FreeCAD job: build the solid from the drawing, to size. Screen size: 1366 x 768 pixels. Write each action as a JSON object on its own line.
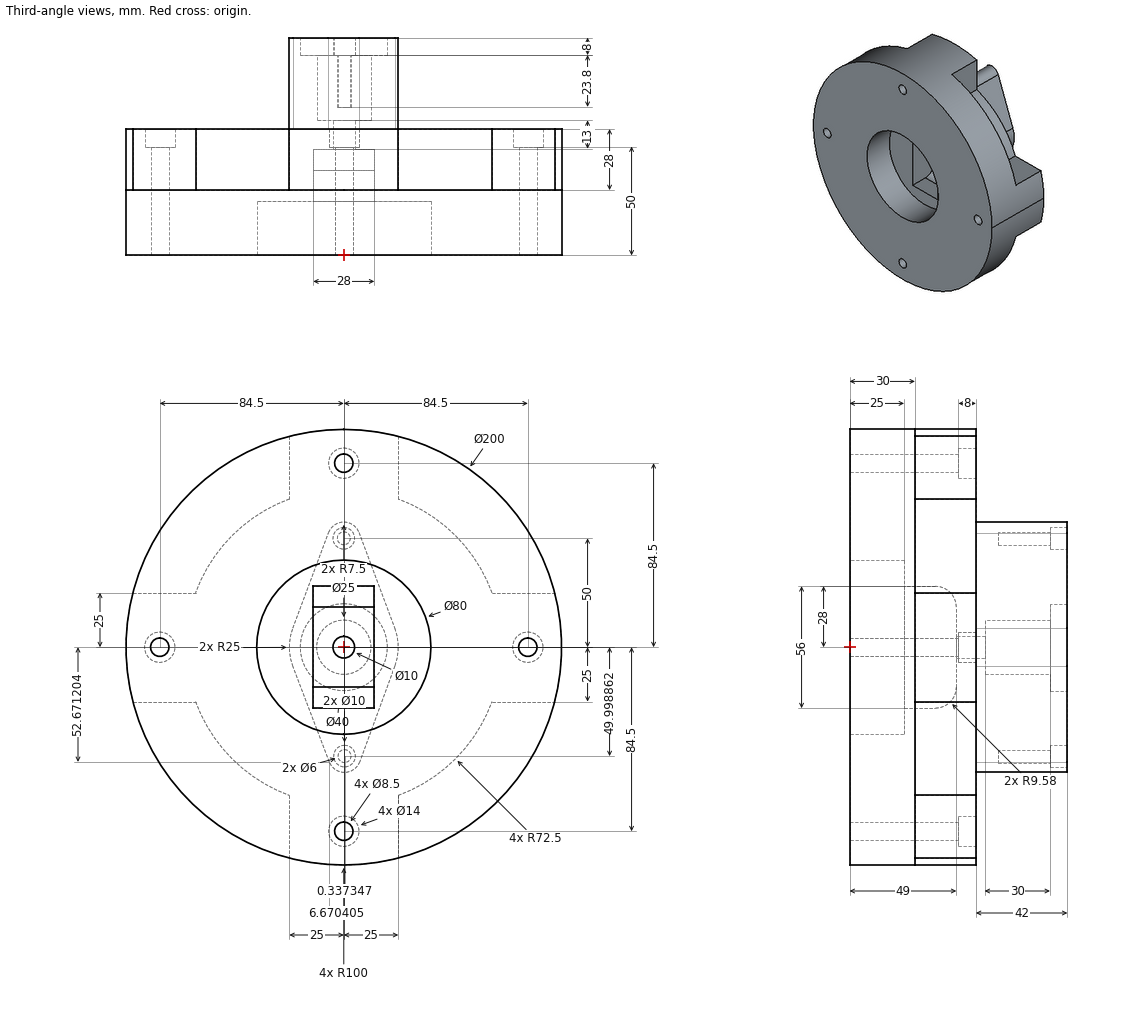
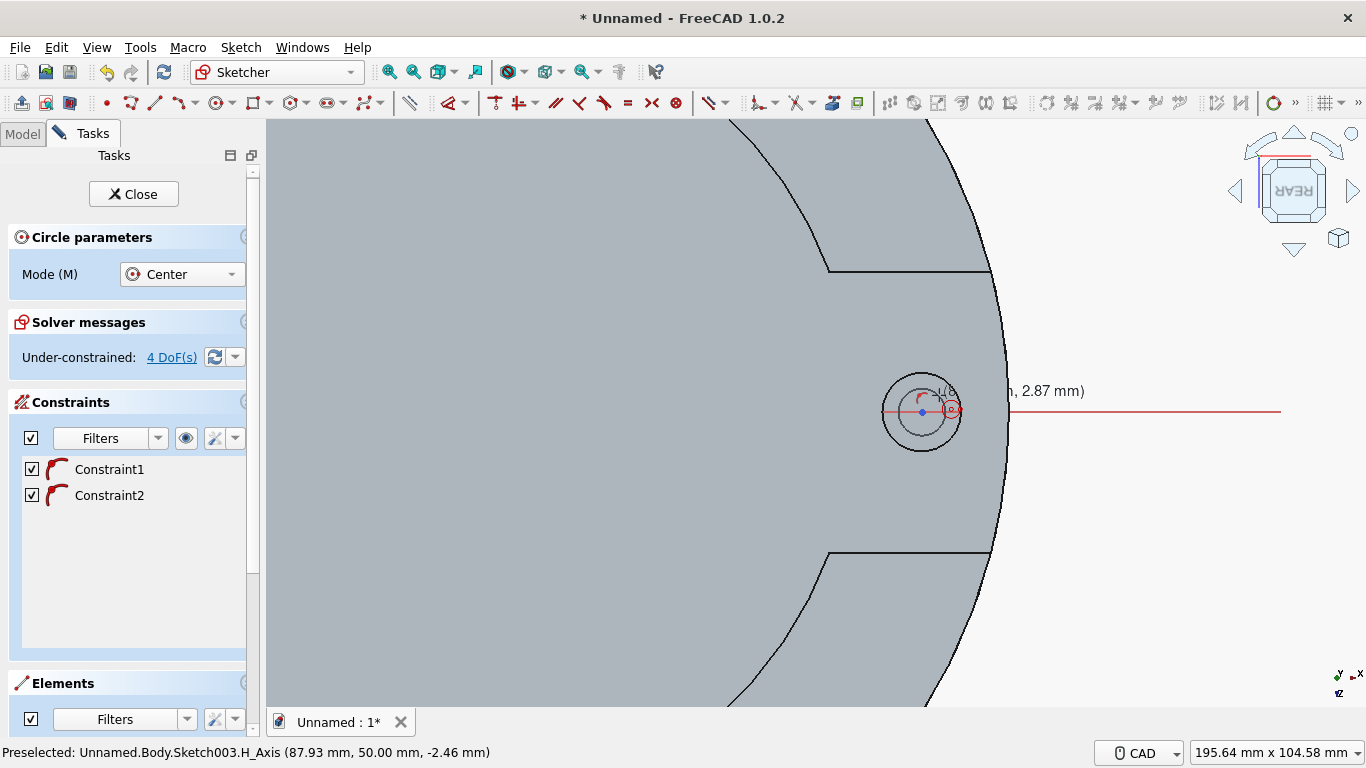
{"action": "scroll", "coordinate": [923, 414], "scroll_direction": "down", "scroll_amount": 5}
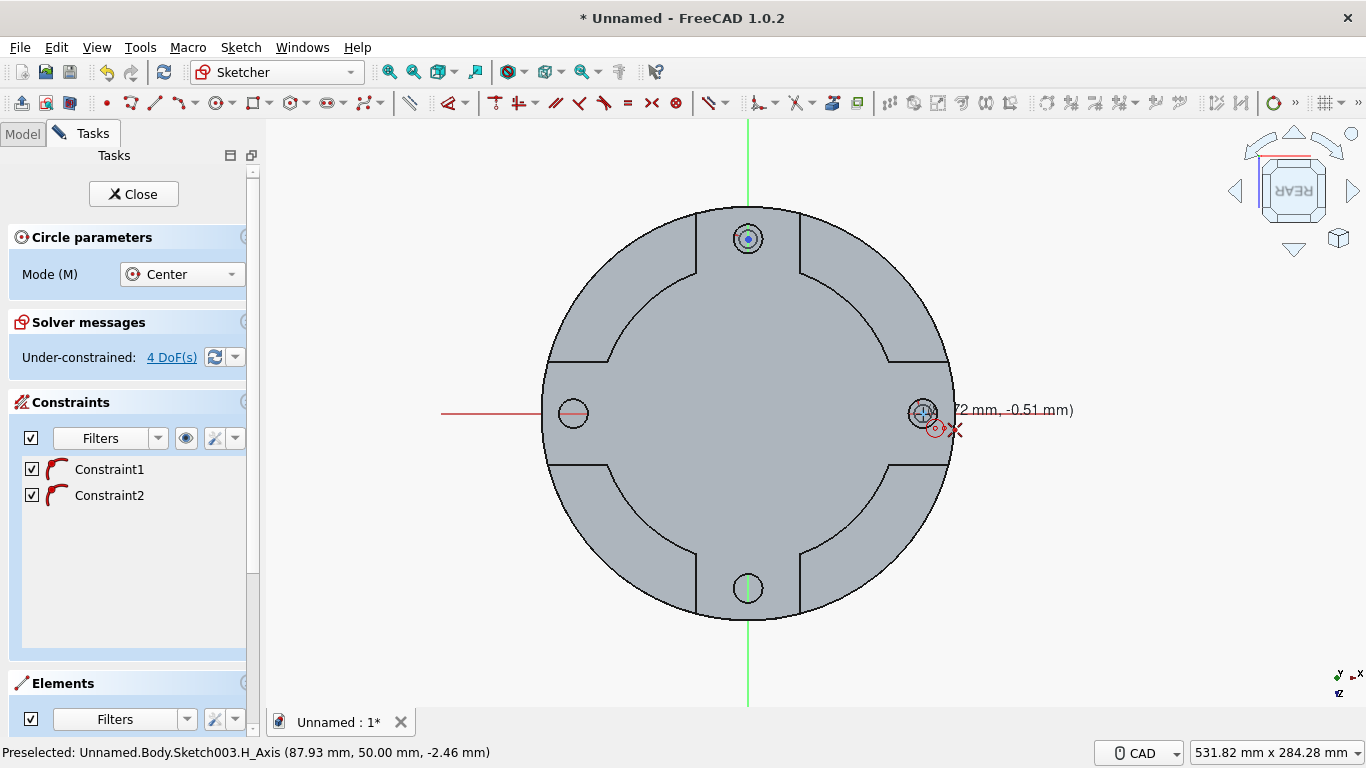
{"action": "scroll", "coordinate": [748, 588], "scroll_direction": "up", "scroll_amount": 5}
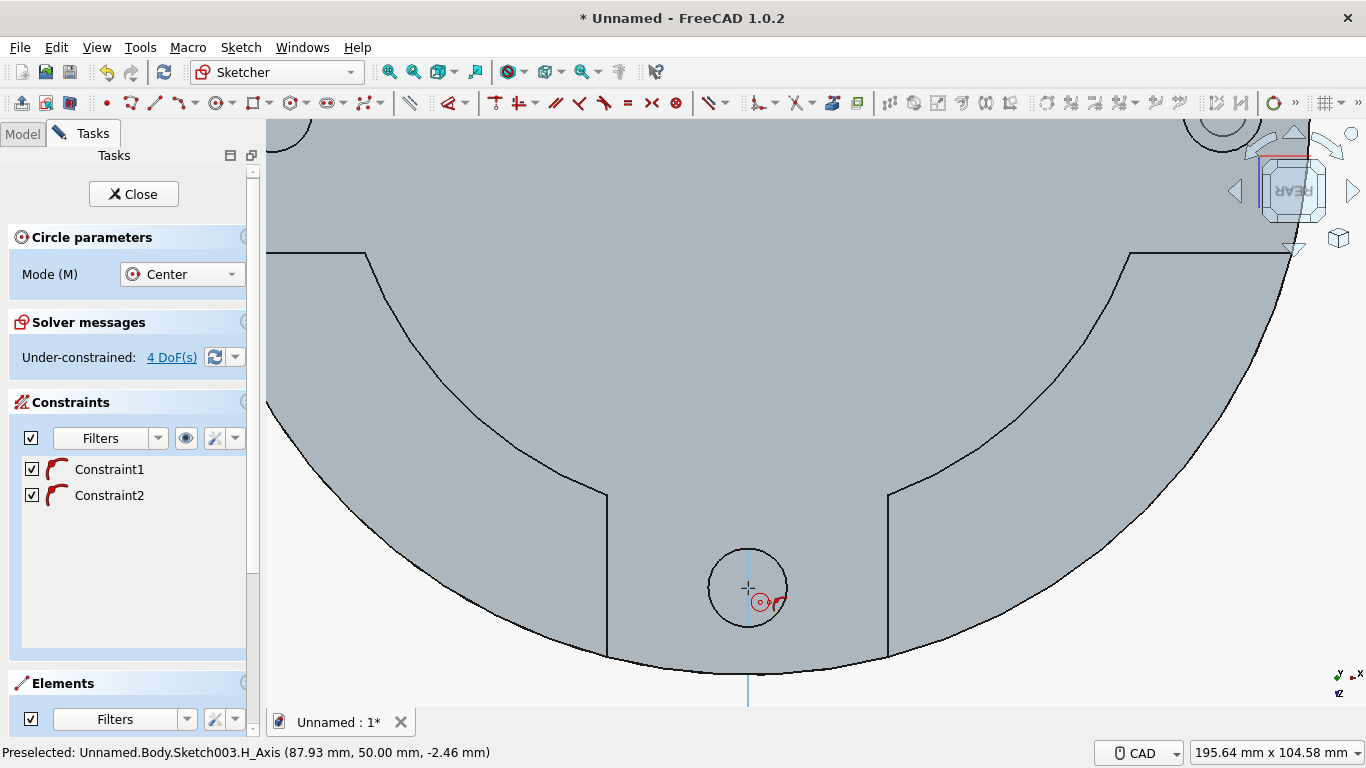
{"action": "left_click", "coordinate": [748, 588]}
{"action": "left_click", "coordinate": [765, 571]}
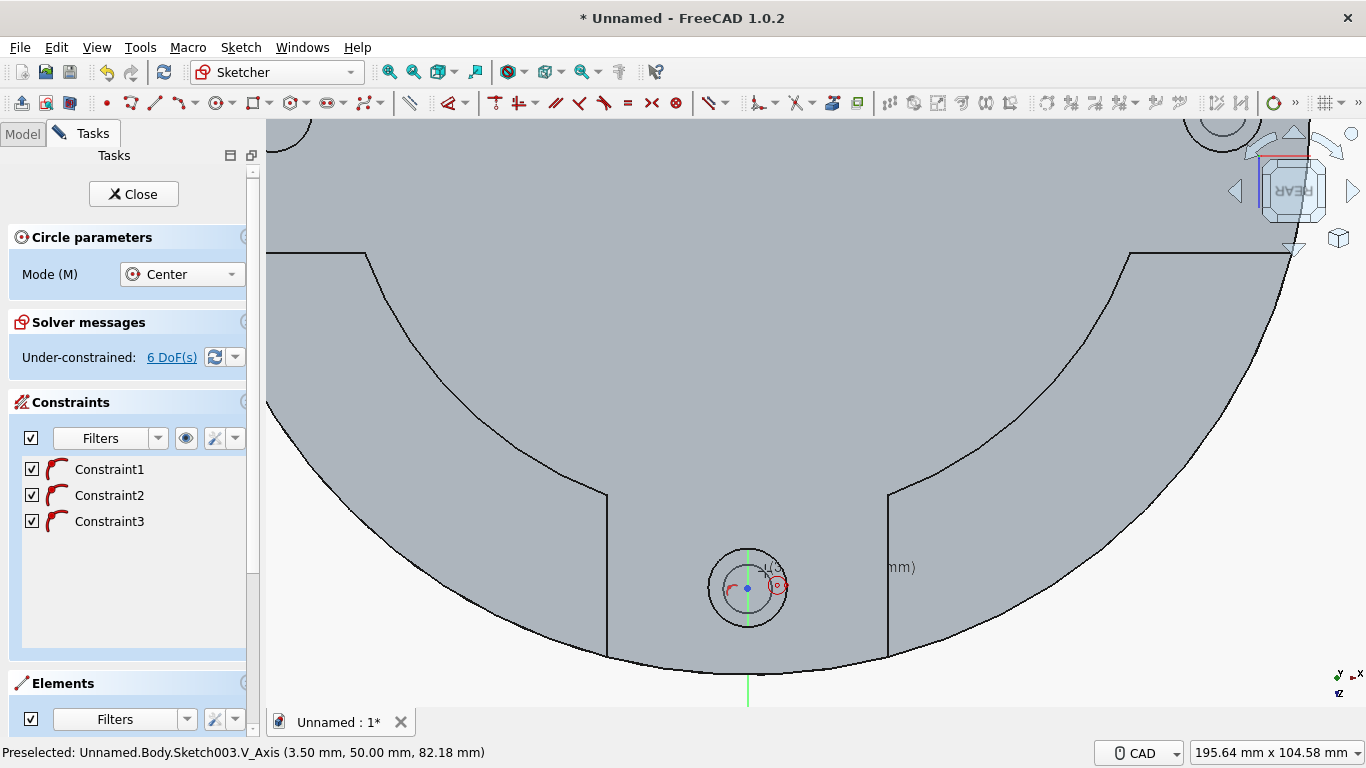
{"action": "scroll", "coordinate": [747, 588], "scroll_direction": "down", "scroll_amount": 5}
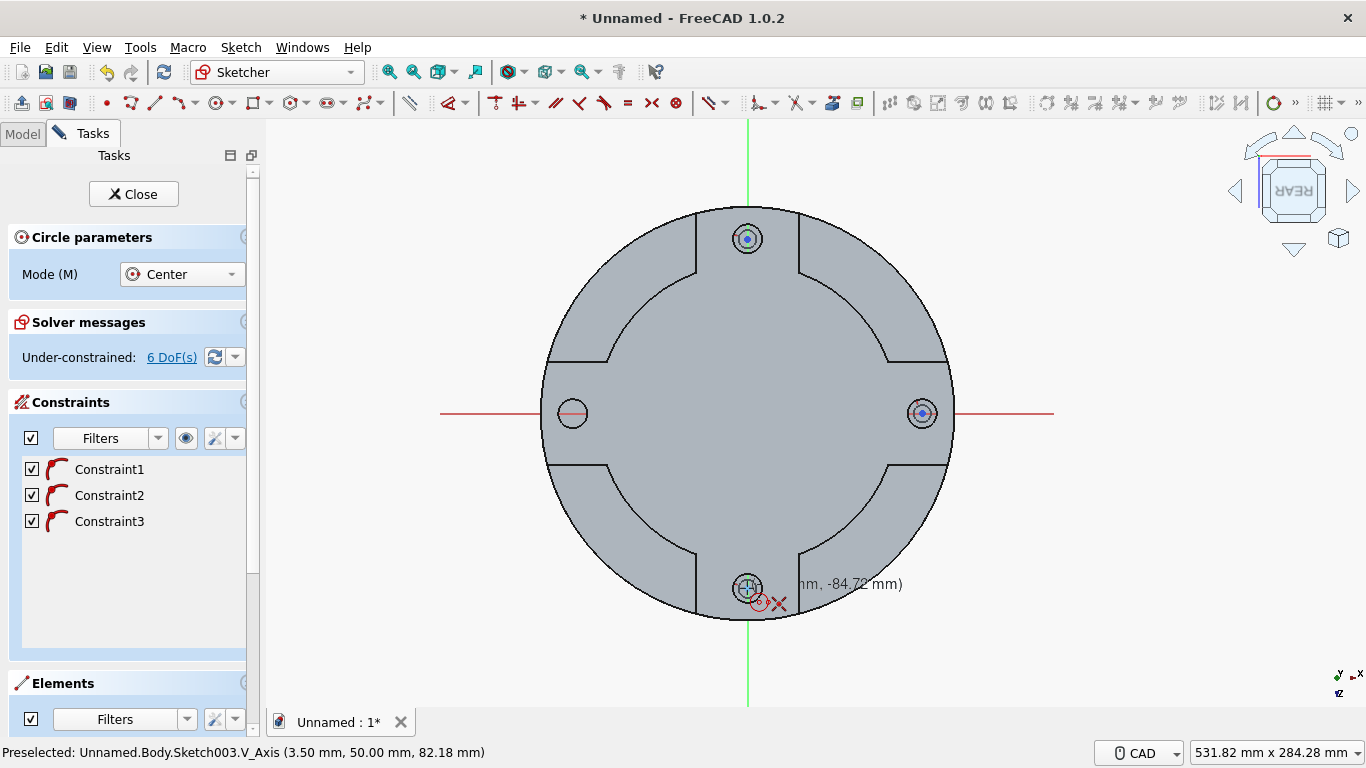
{"action": "scroll", "coordinate": [573, 414], "scroll_direction": "up", "scroll_amount": 5}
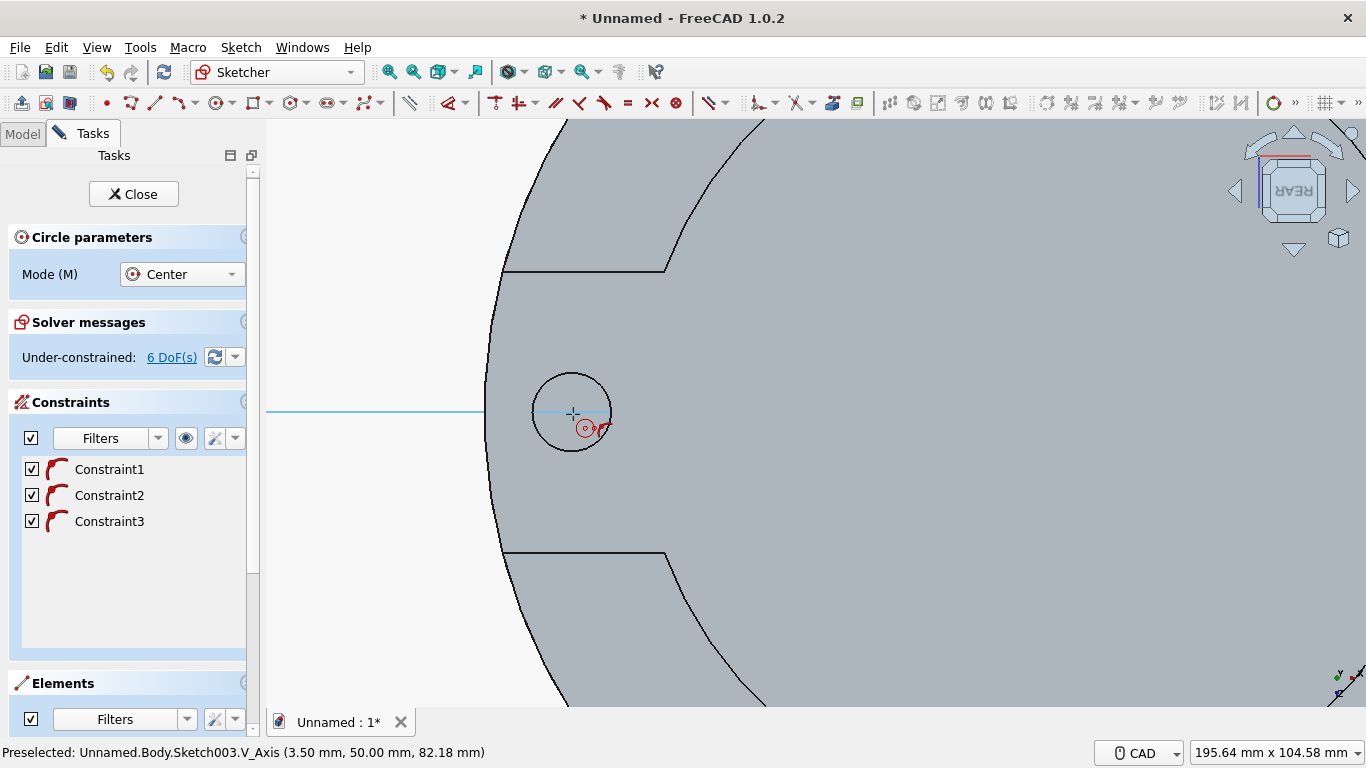
{"action": "left_click", "coordinate": [572, 412]}
{"action": "left_click", "coordinate": [589, 395]}
{"action": "key", "text": "Escape"}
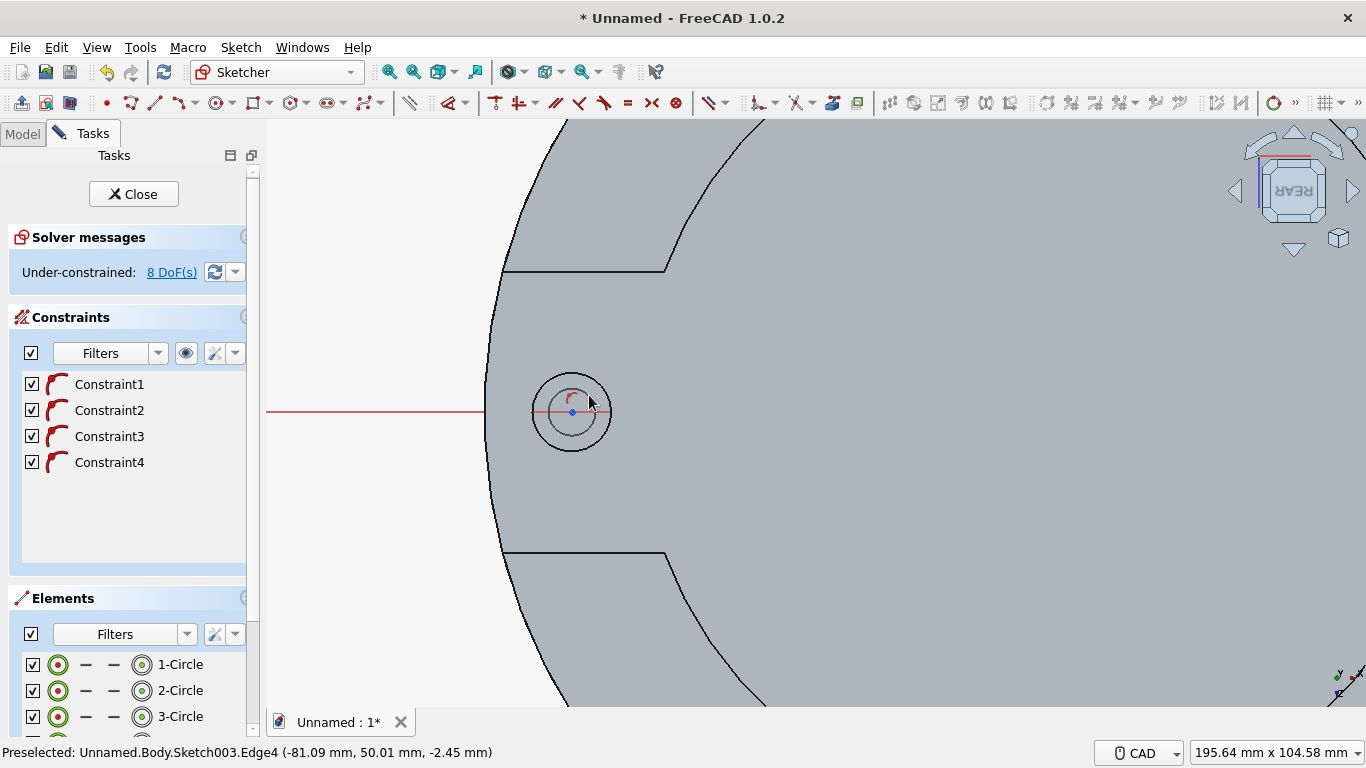
{"action": "scroll", "coordinate": [573, 414], "scroll_direction": "down", "scroll_amount": 5}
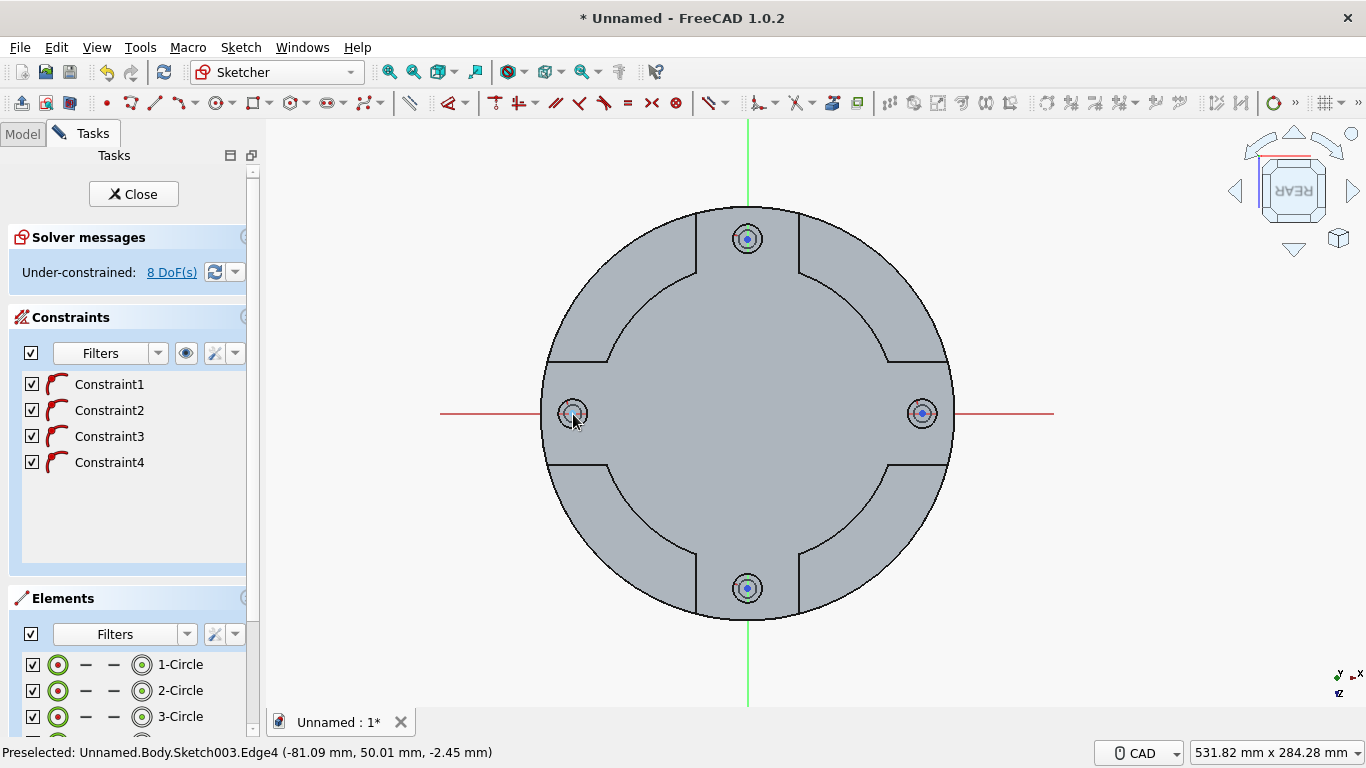
{"action": "scroll", "coordinate": [754, 233], "scroll_direction": "up", "scroll_amount": 4}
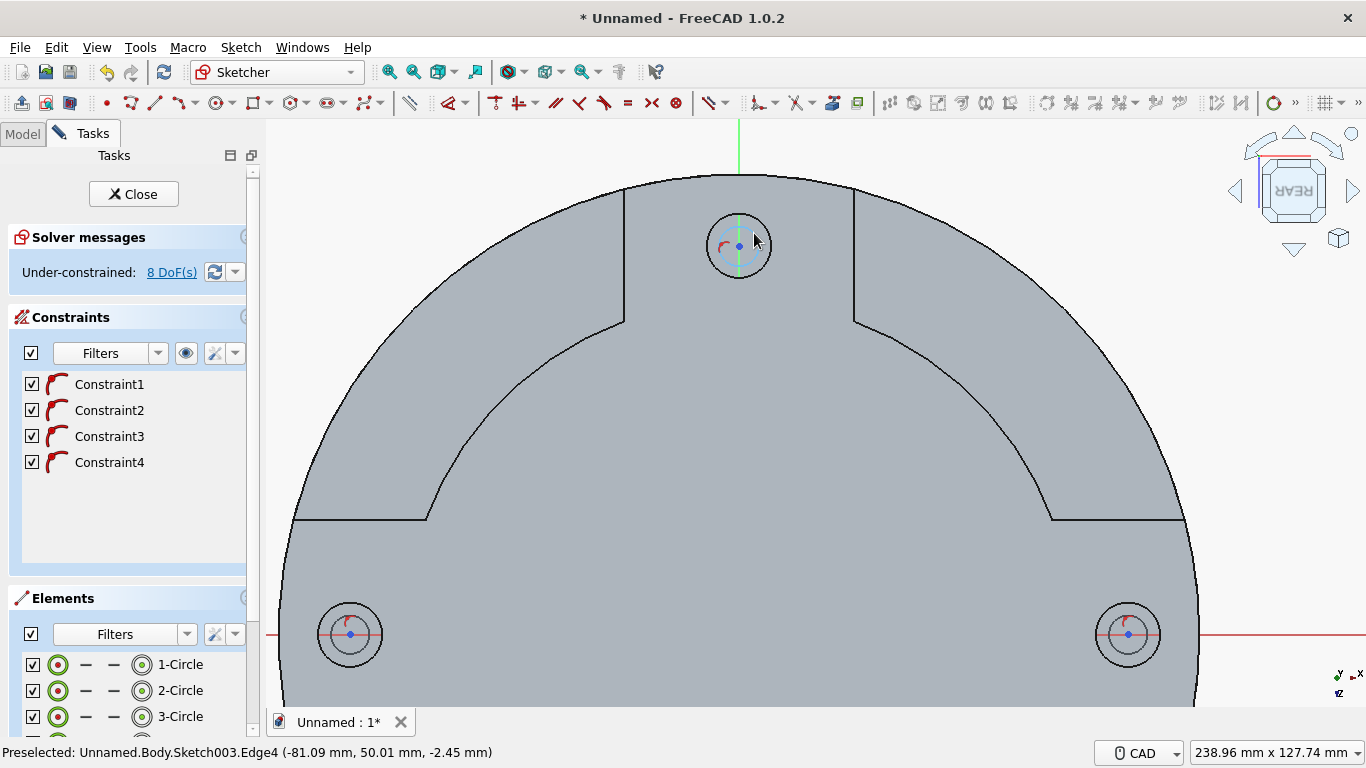
{"action": "left_click", "coordinate": [753, 232]}